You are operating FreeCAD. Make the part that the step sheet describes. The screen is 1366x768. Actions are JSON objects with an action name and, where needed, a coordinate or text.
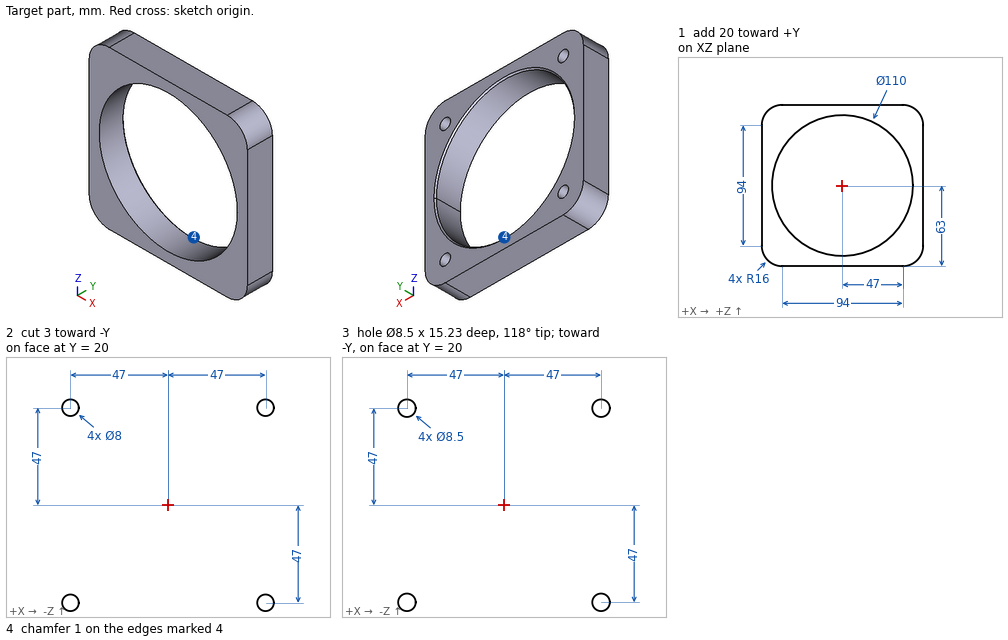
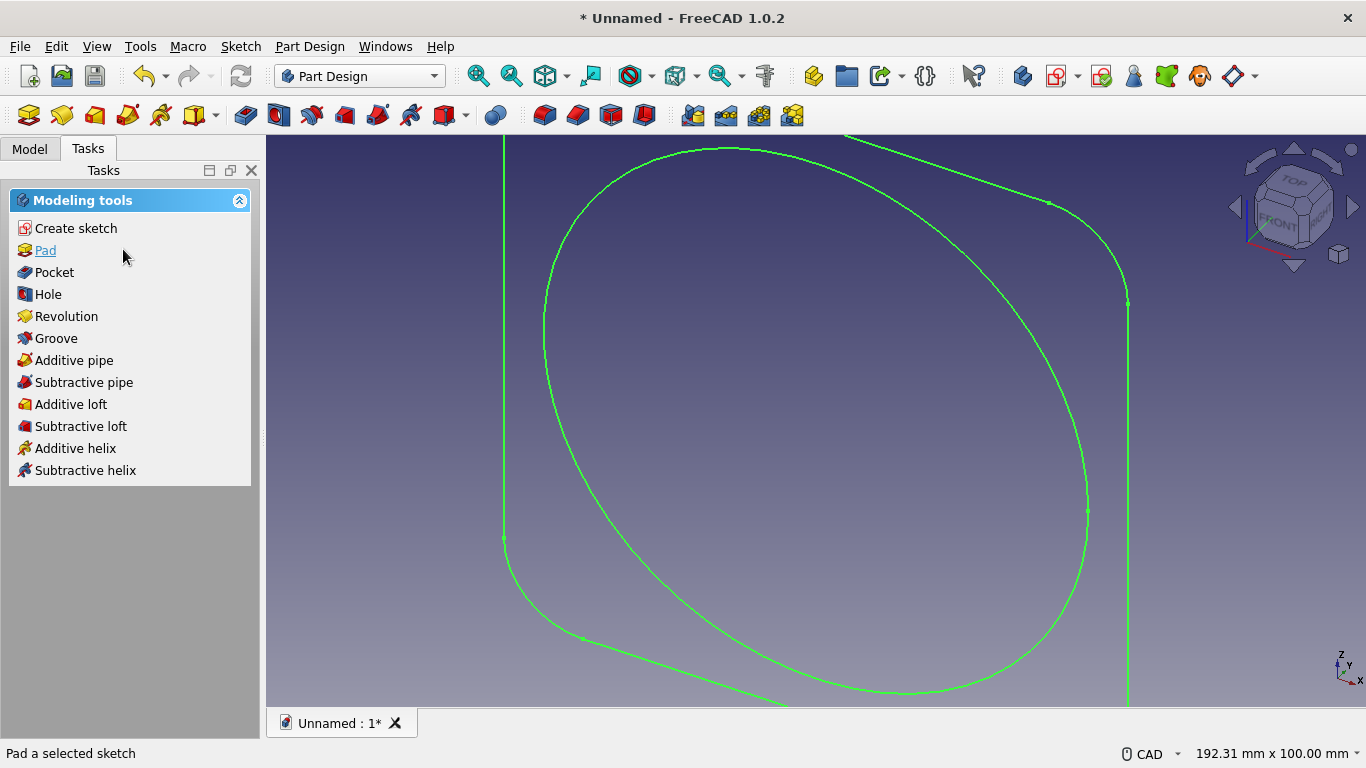
{"action": "left_click", "coordinate": [29, 116]}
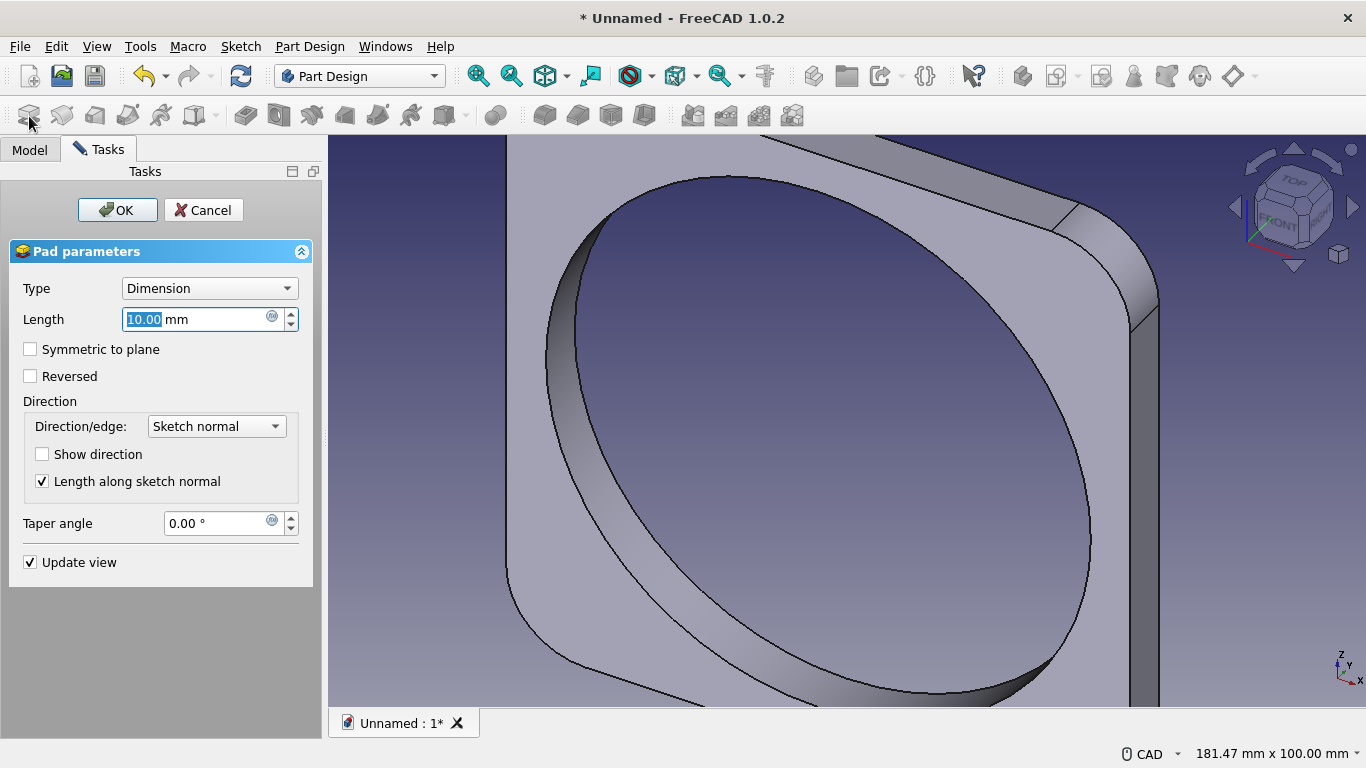
{"action": "type", "text": "20"}
{"action": "key", "text": "Tab"}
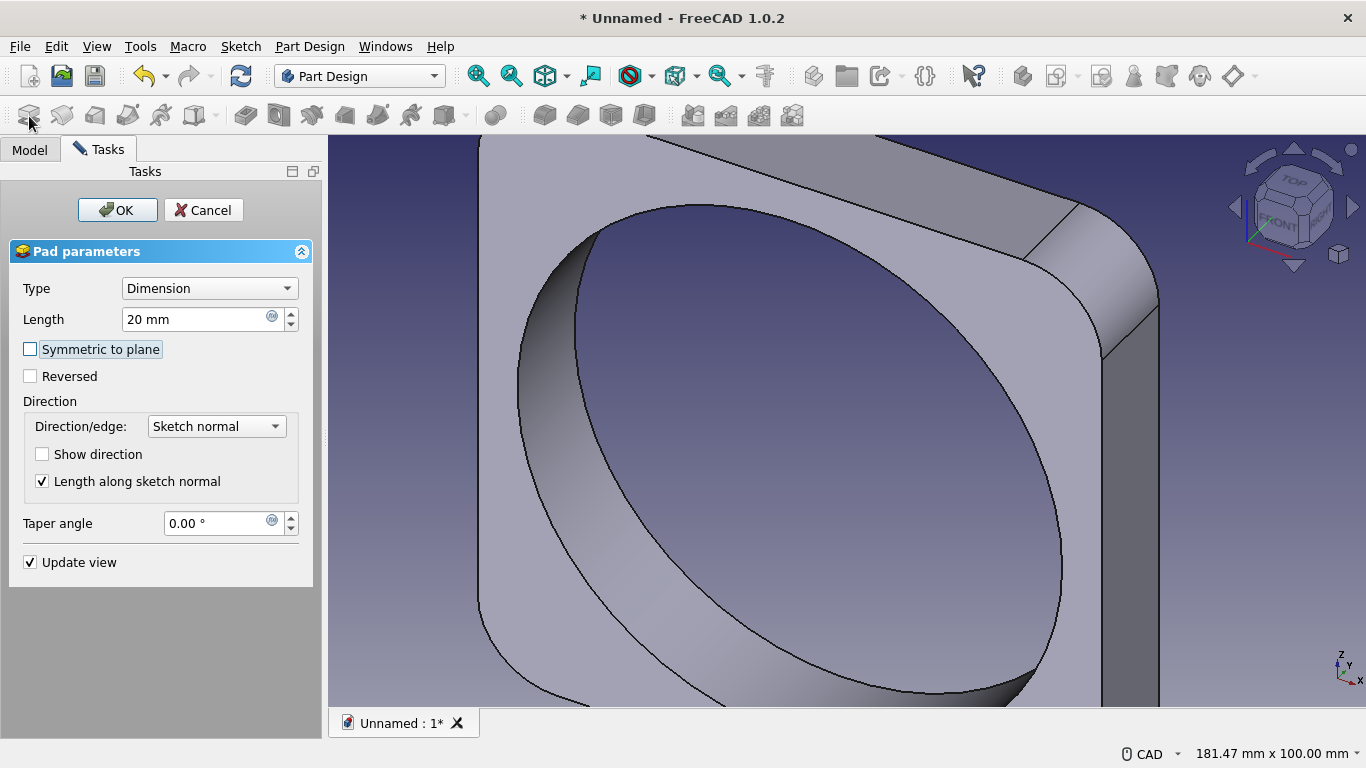
{"action": "left_click", "coordinate": [31, 376]}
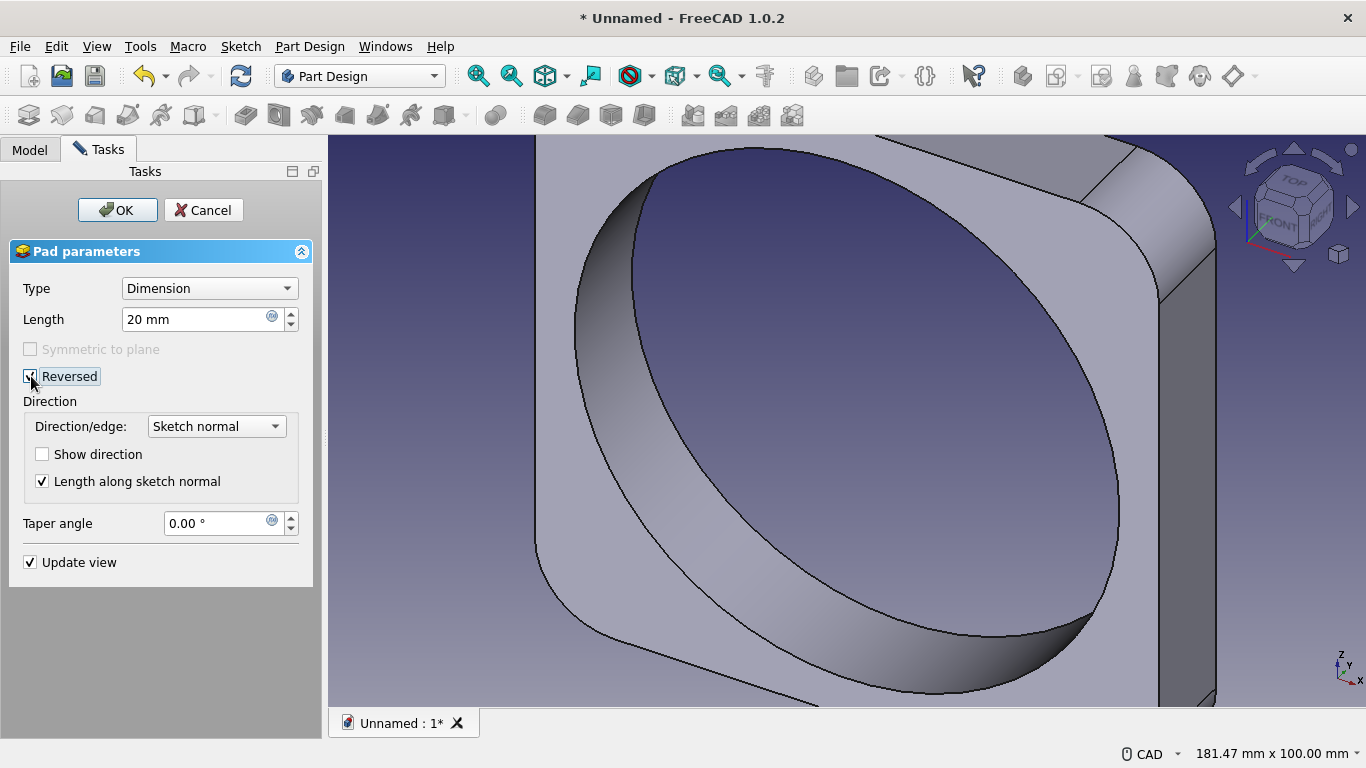
{"action": "left_click", "coordinate": [118, 210]}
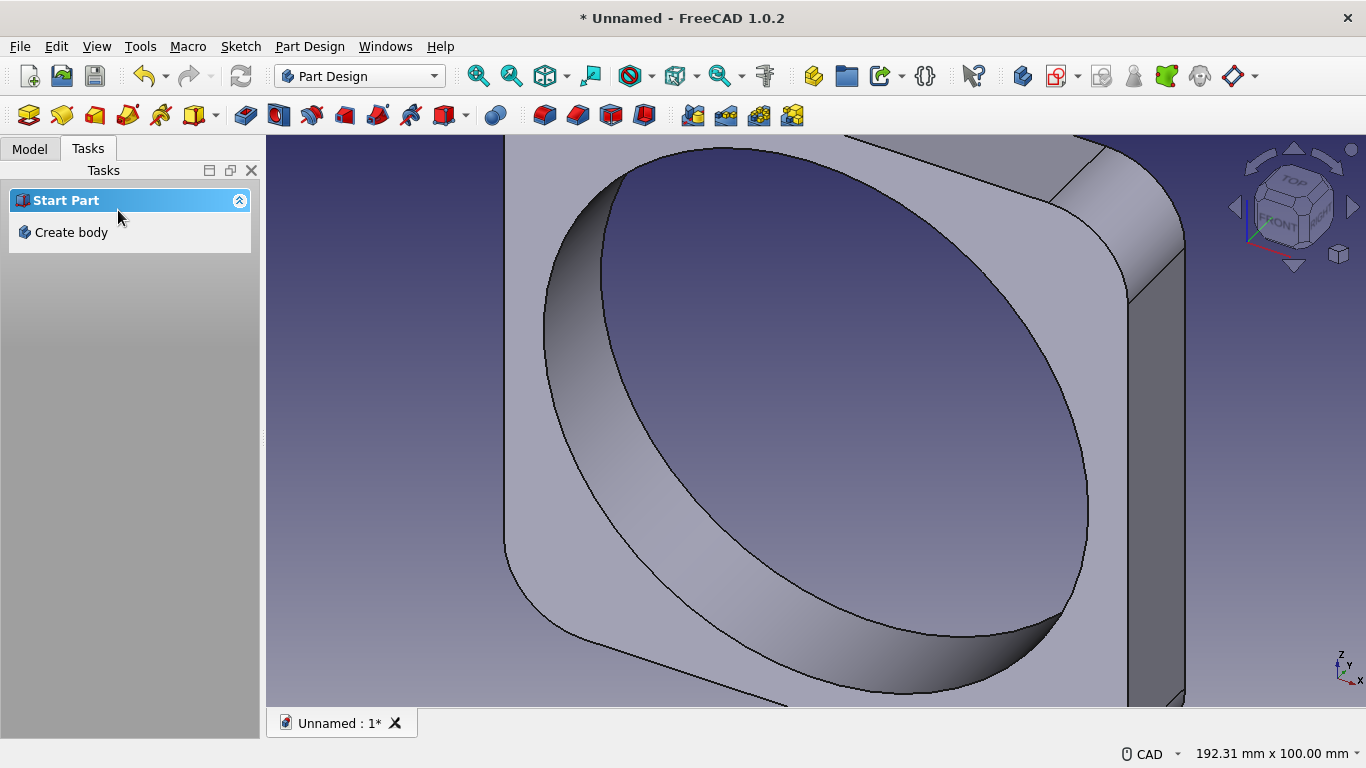
{"action": "key", "text": "v f"}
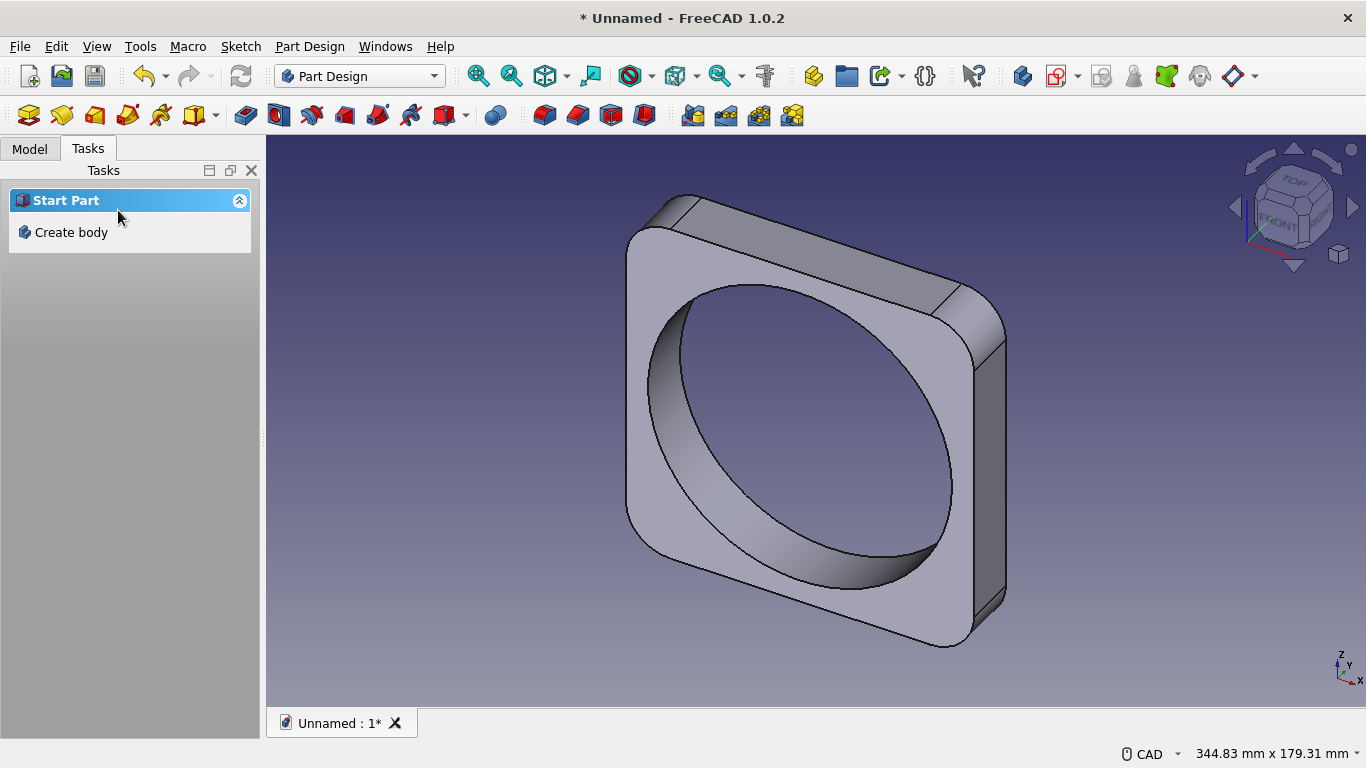
{"action": "key", "text": "4"}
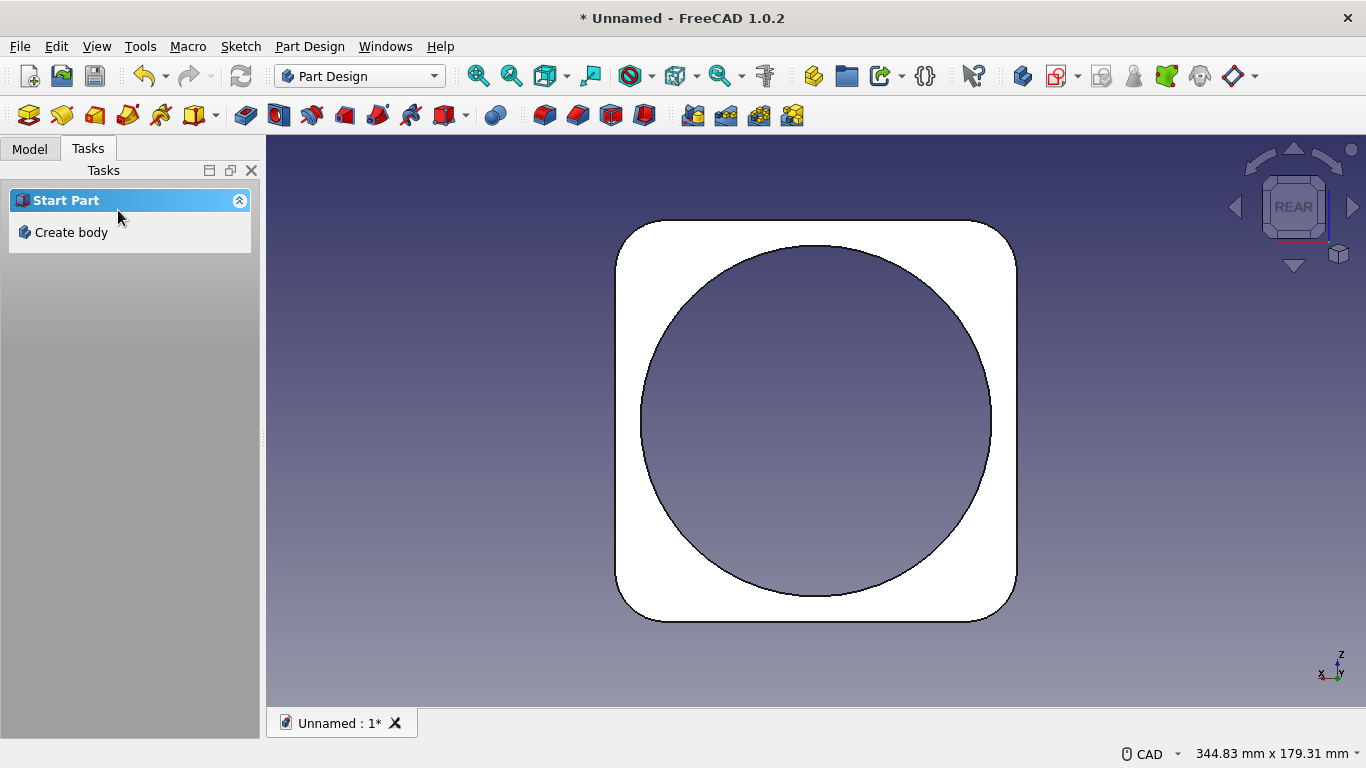
{"action": "left_click", "coordinate": [644, 305]}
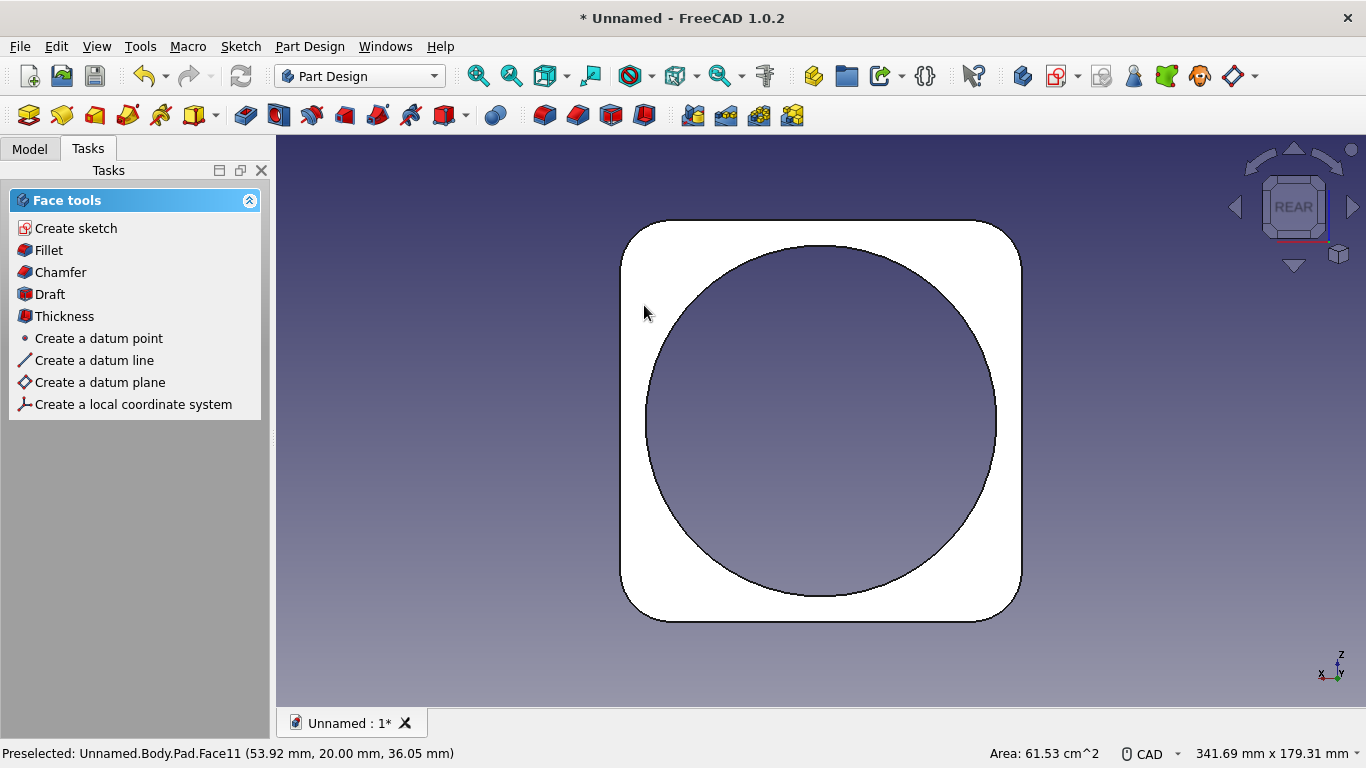
{"action": "left_click", "coordinate": [1056, 76]}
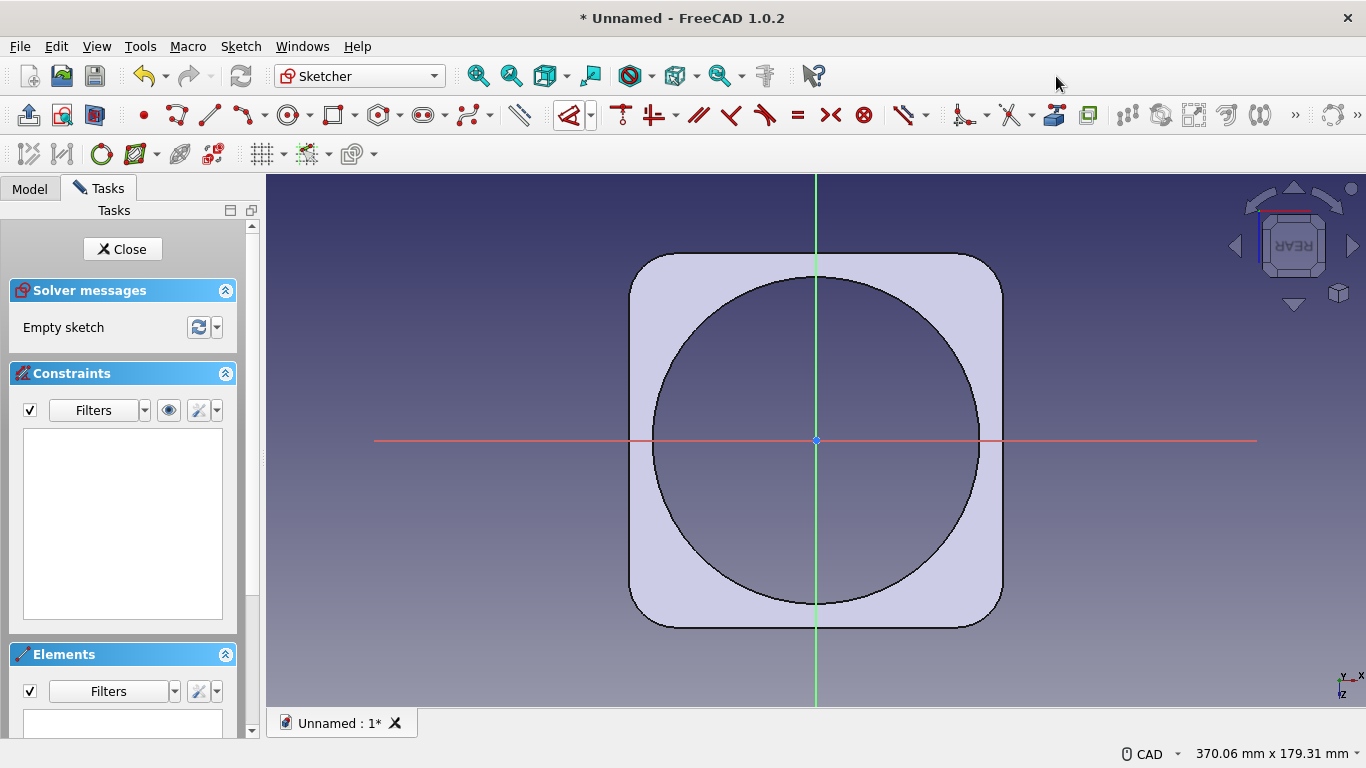
{"action": "left_click", "coordinate": [288, 116]}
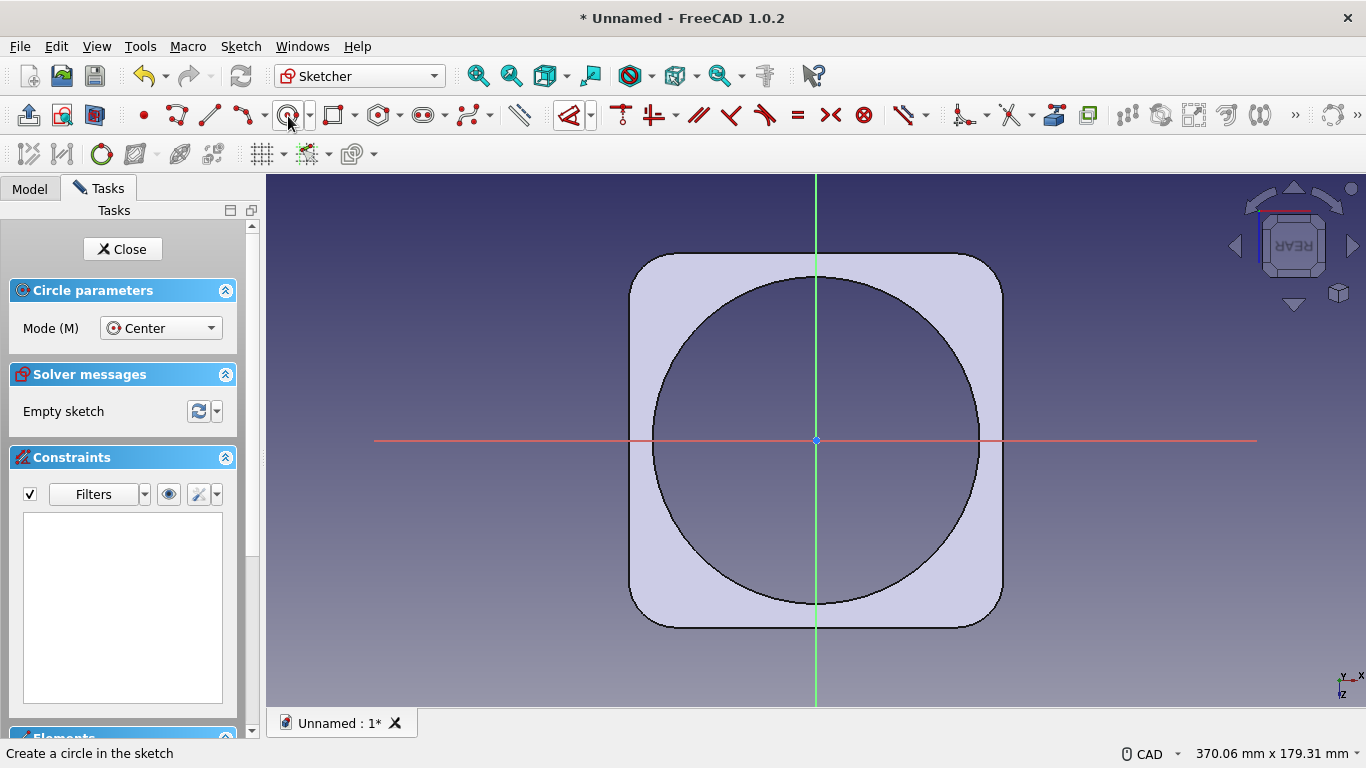
{"action": "scroll", "coordinate": [676, 301], "scroll_direction": "up", "scroll_amount": 4}